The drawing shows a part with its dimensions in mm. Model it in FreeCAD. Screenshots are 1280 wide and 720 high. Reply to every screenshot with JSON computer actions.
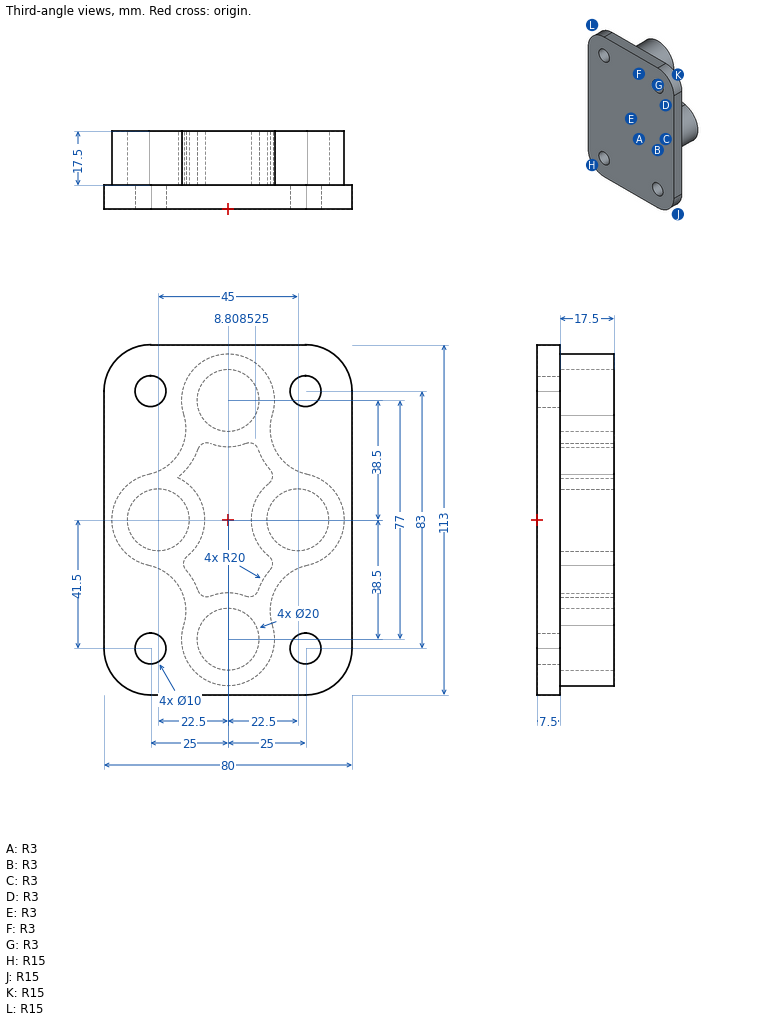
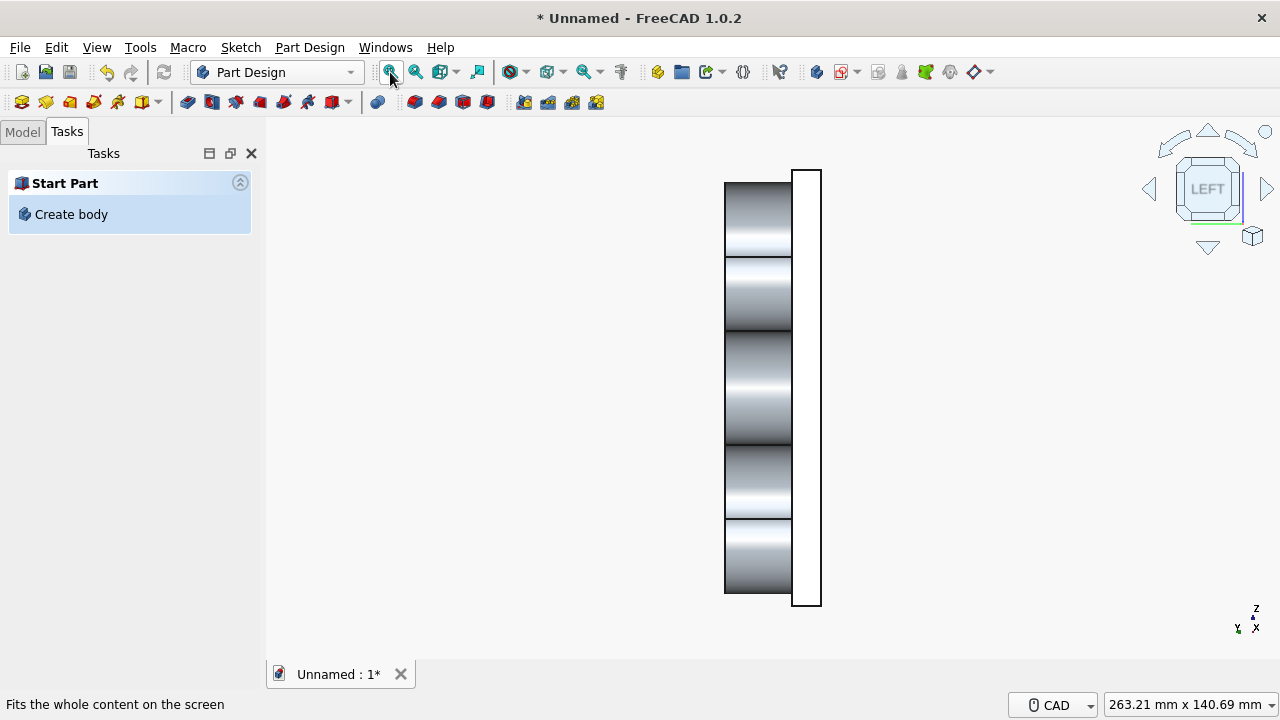
{"action": "key", "text": "v 3"}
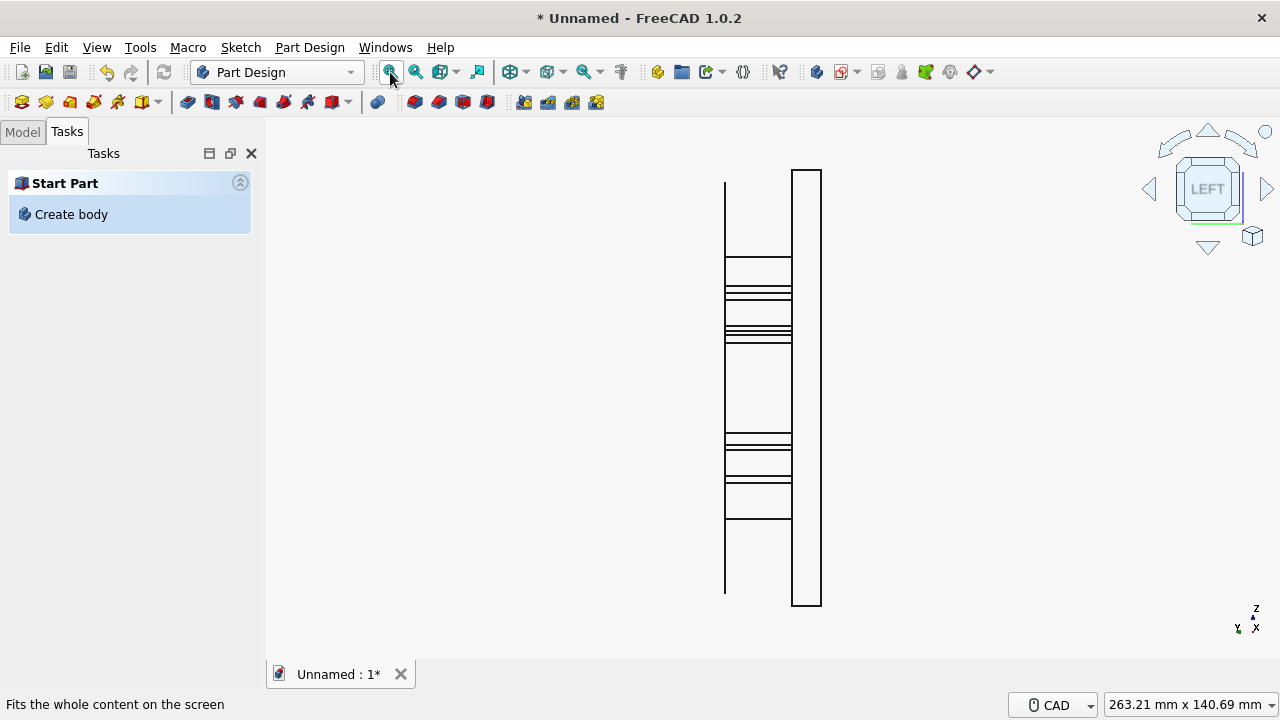
{"action": "key", "text": "0"}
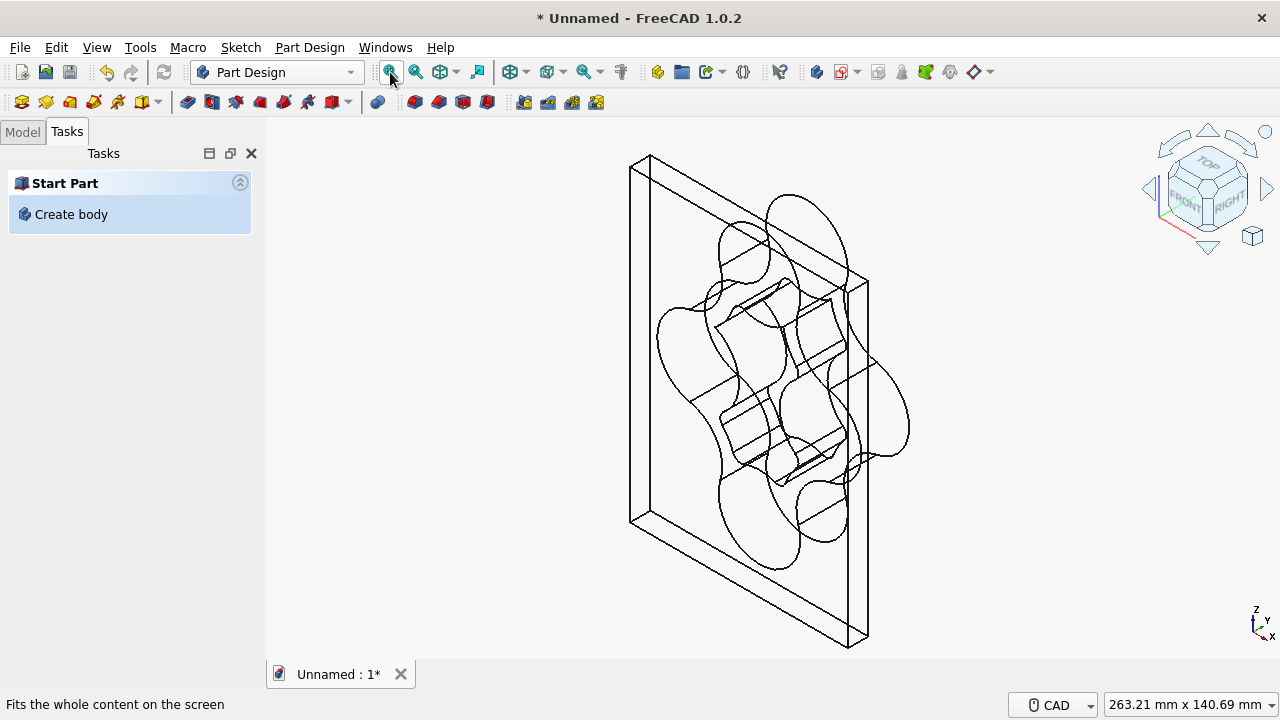
{"action": "key", "text": "2"}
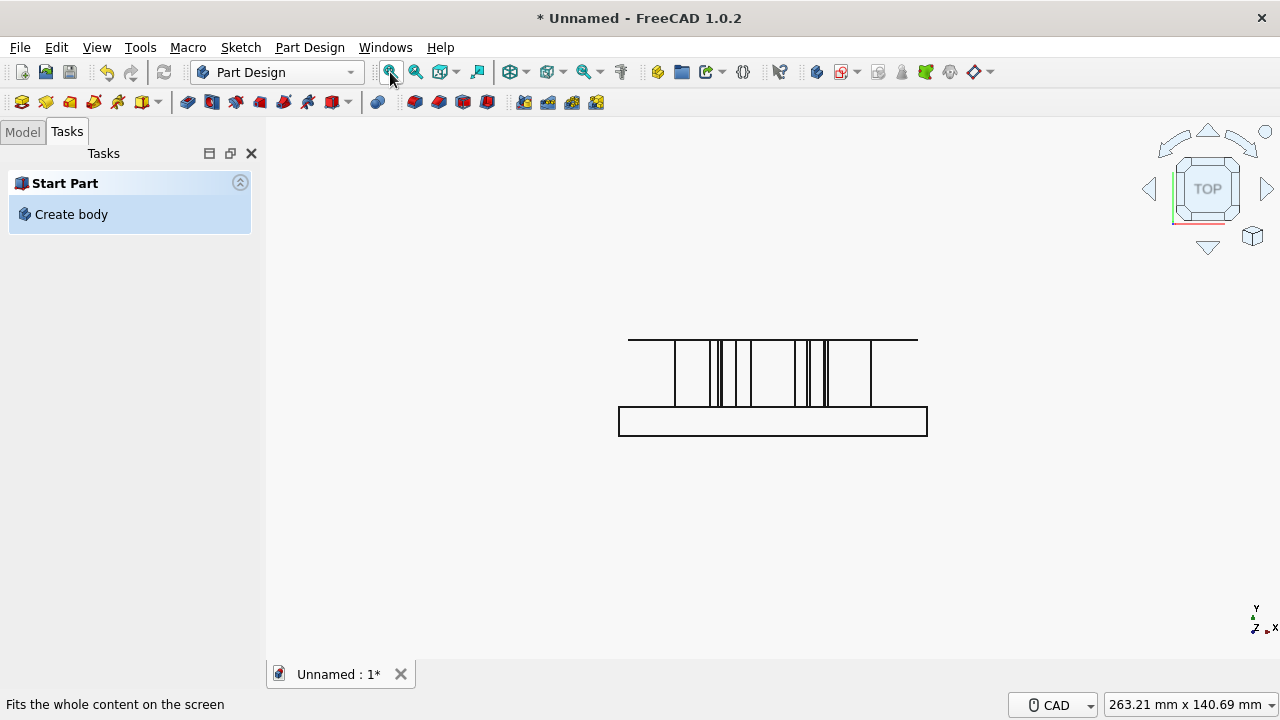
{"action": "key", "text": "v f"}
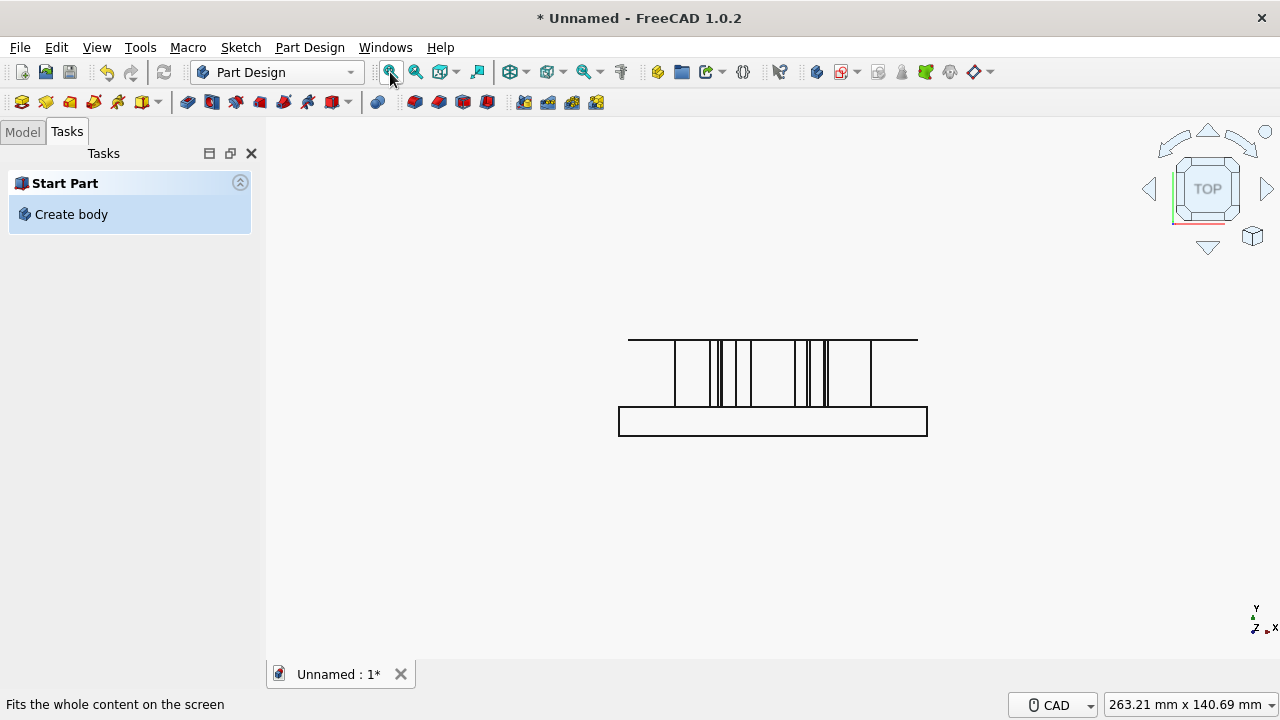
{"action": "left_click", "coordinate": [807, 373]}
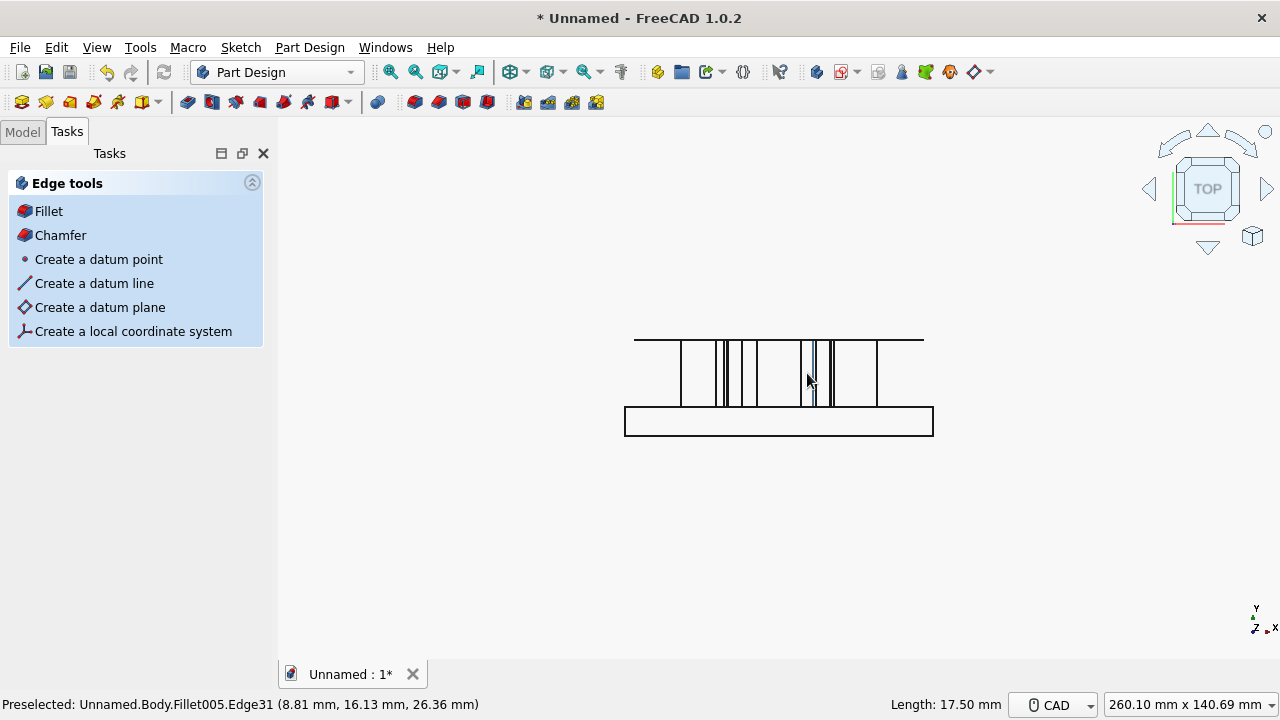
{"action": "key", "text": "v 1"}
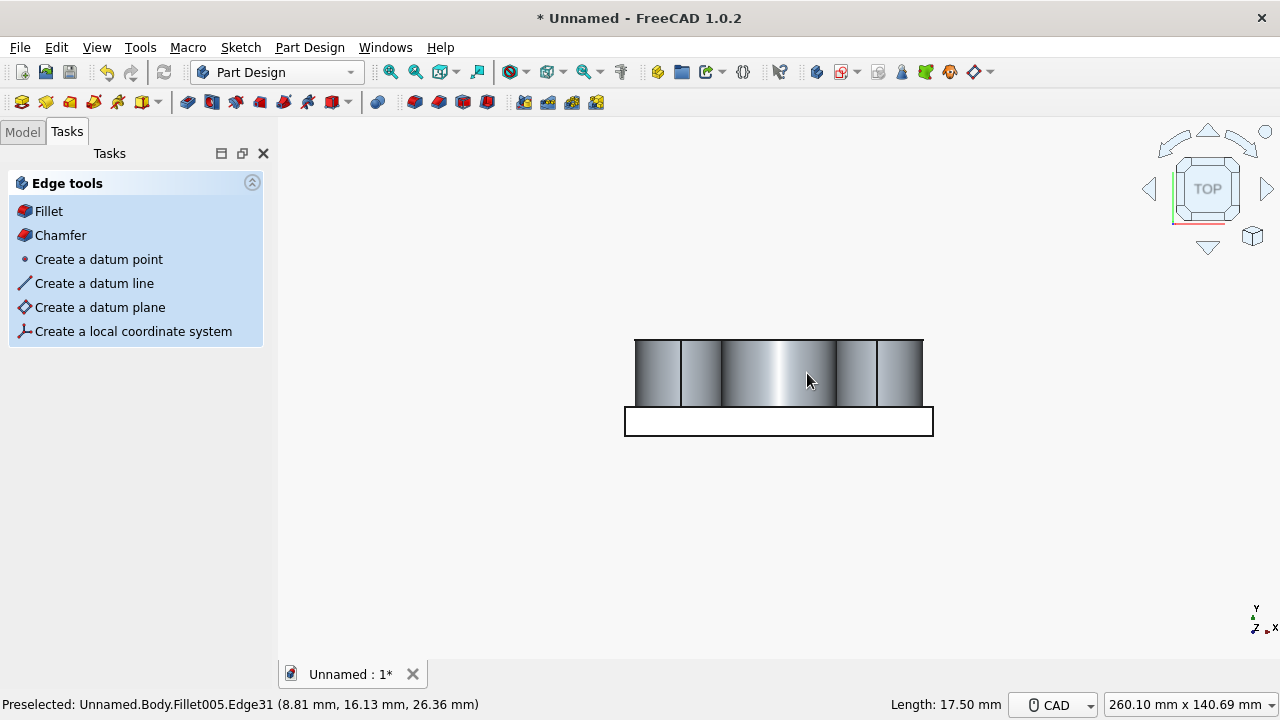
{"action": "left_click", "coordinate": [416, 102]}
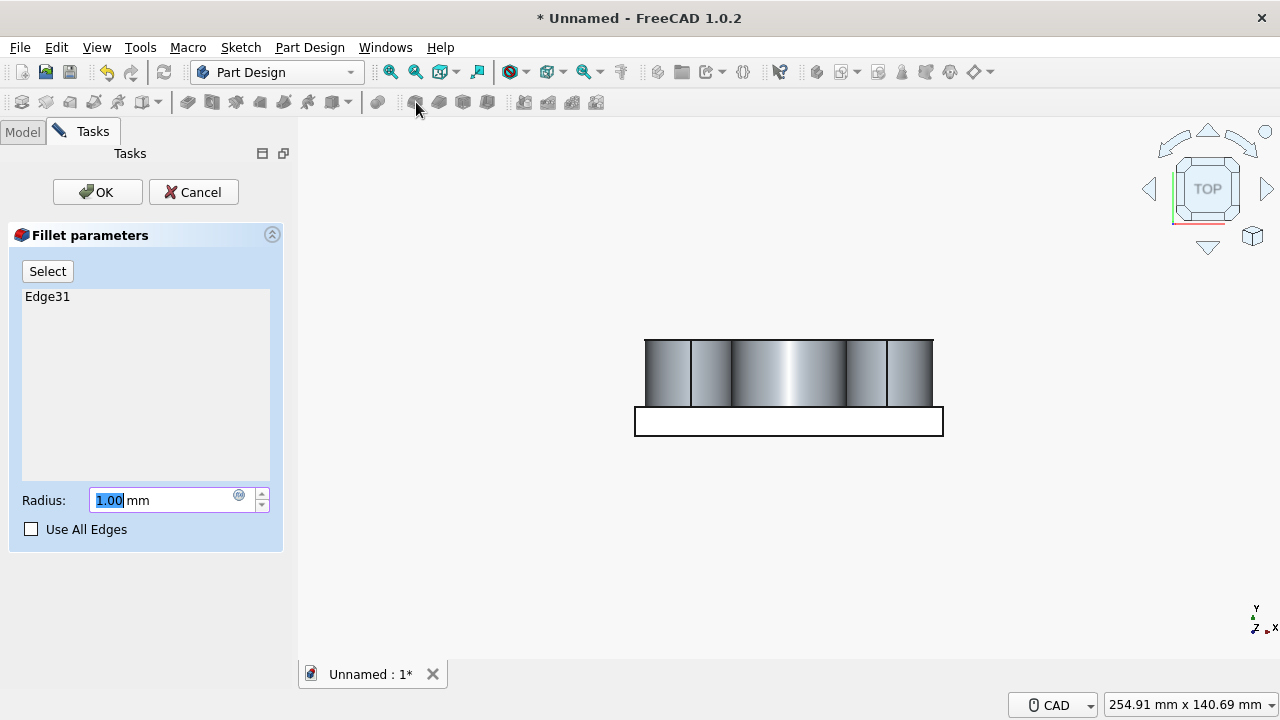
{"action": "type", "text": "3"}
{"action": "key", "text": "Tab"}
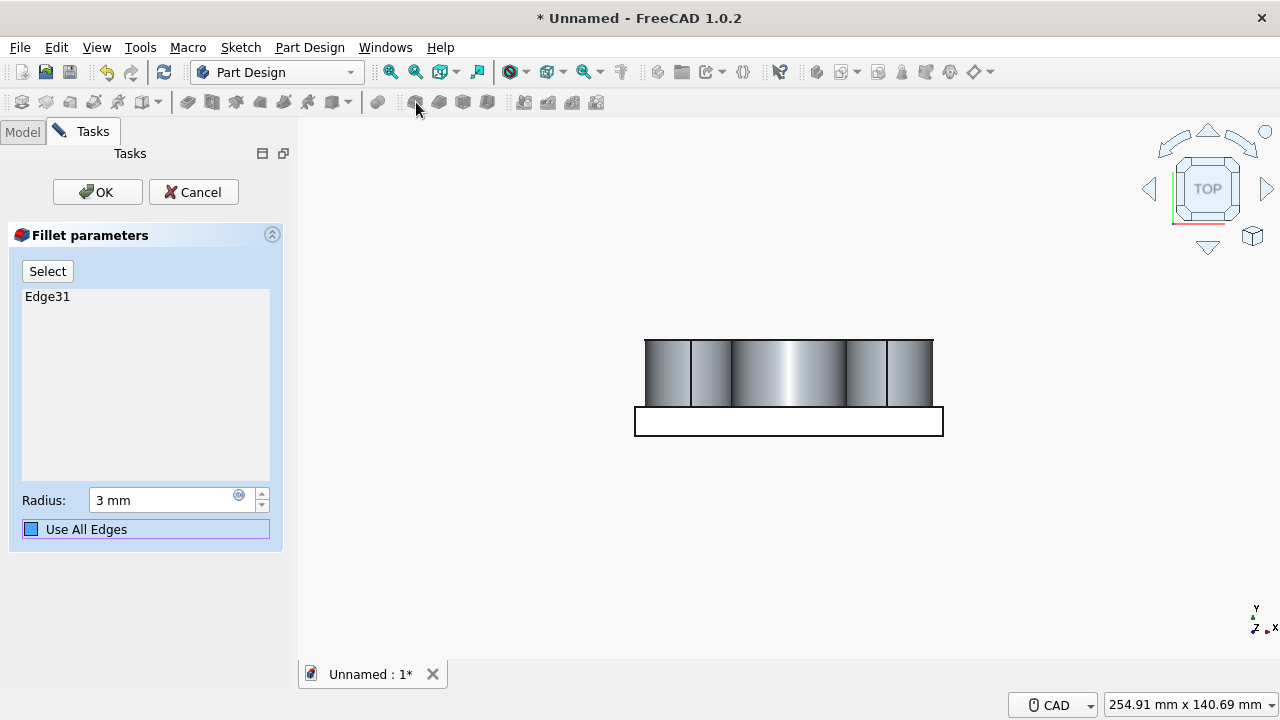
{"action": "left_click", "coordinate": [98, 192]}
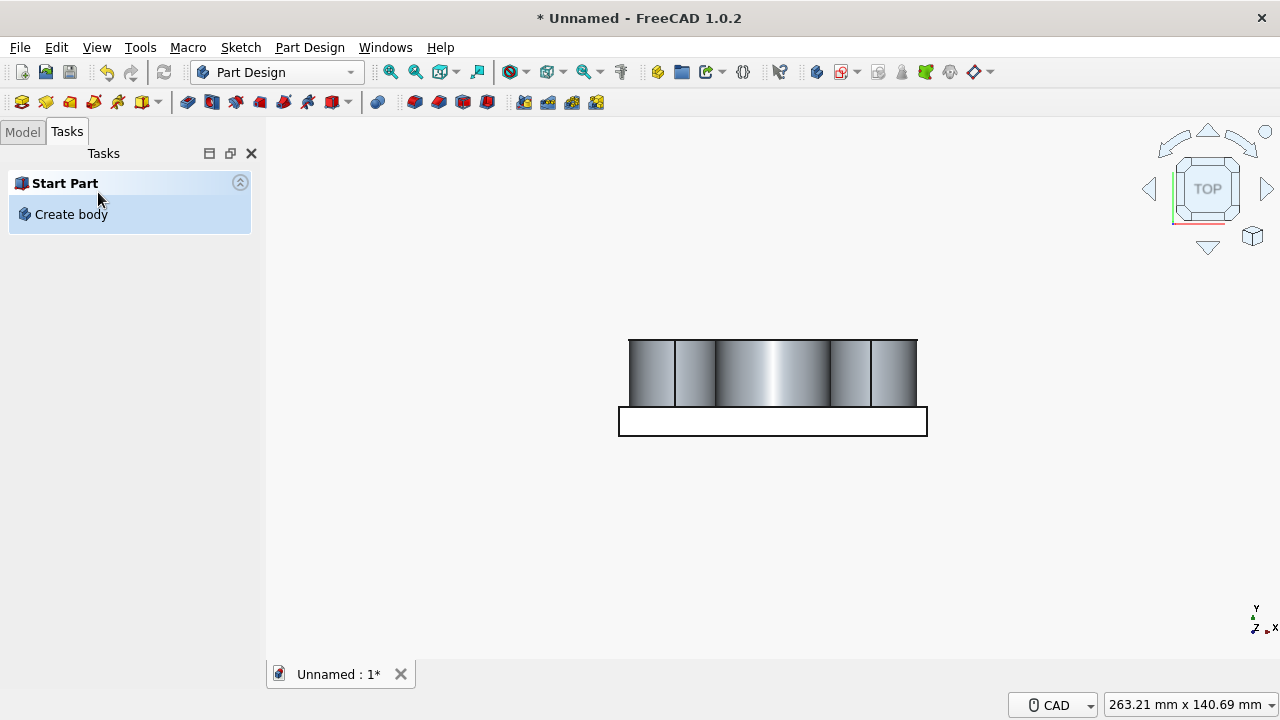
{"action": "key", "text": "v f"}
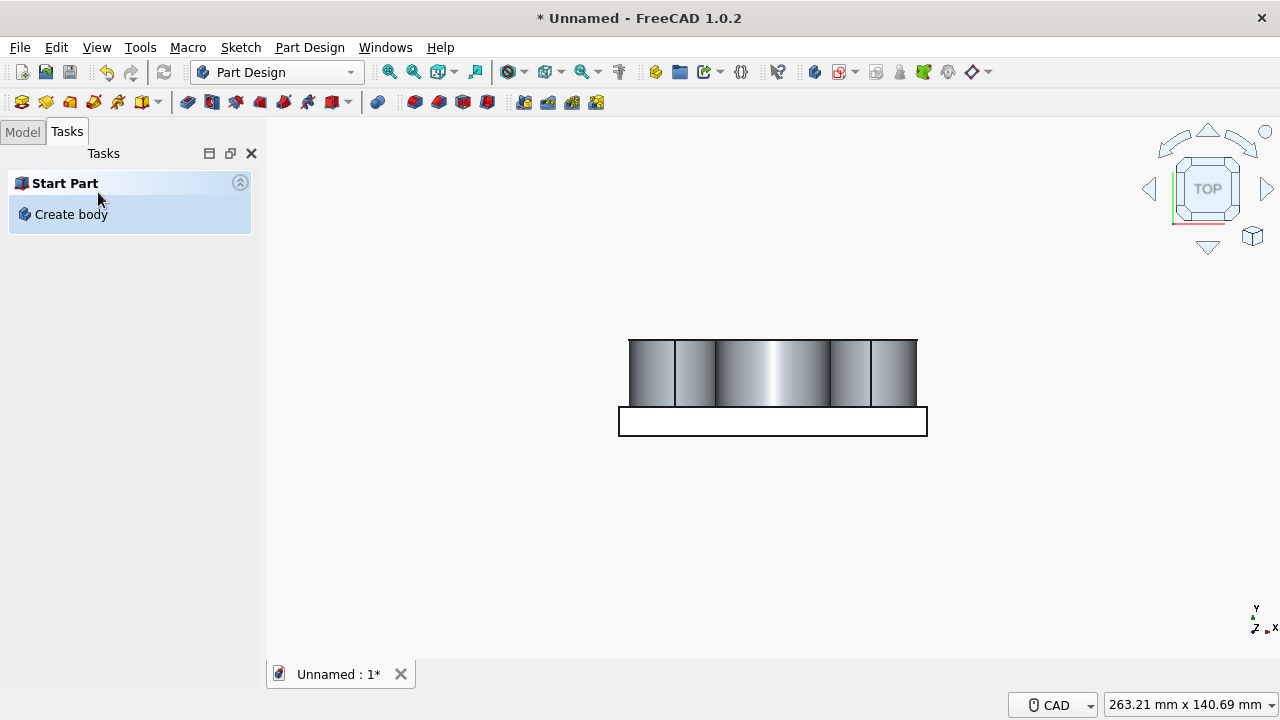
{"action": "key", "text": "4"}